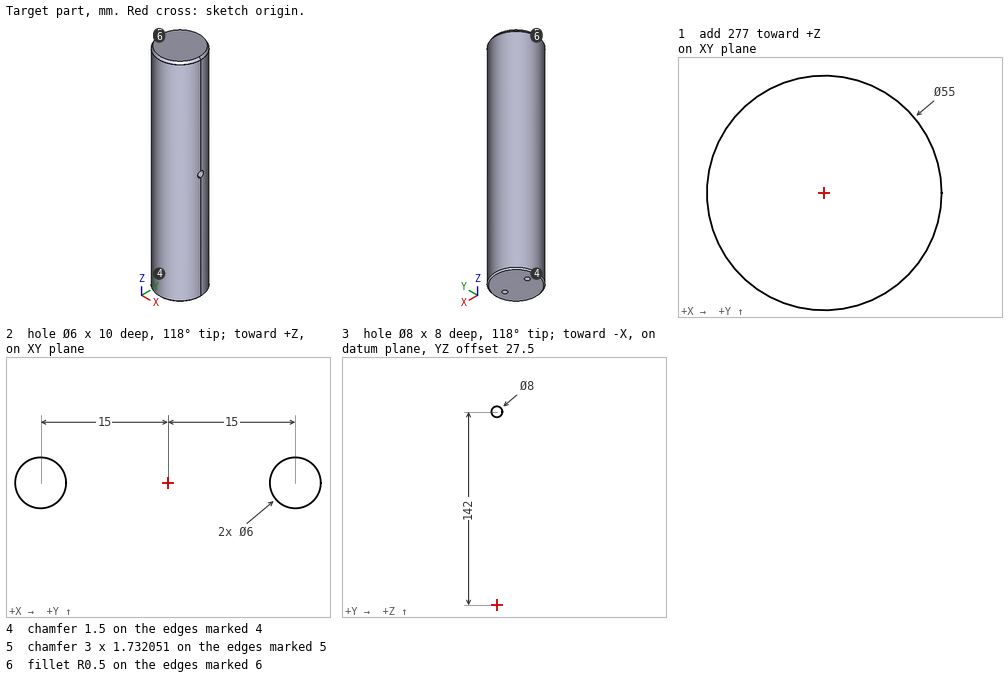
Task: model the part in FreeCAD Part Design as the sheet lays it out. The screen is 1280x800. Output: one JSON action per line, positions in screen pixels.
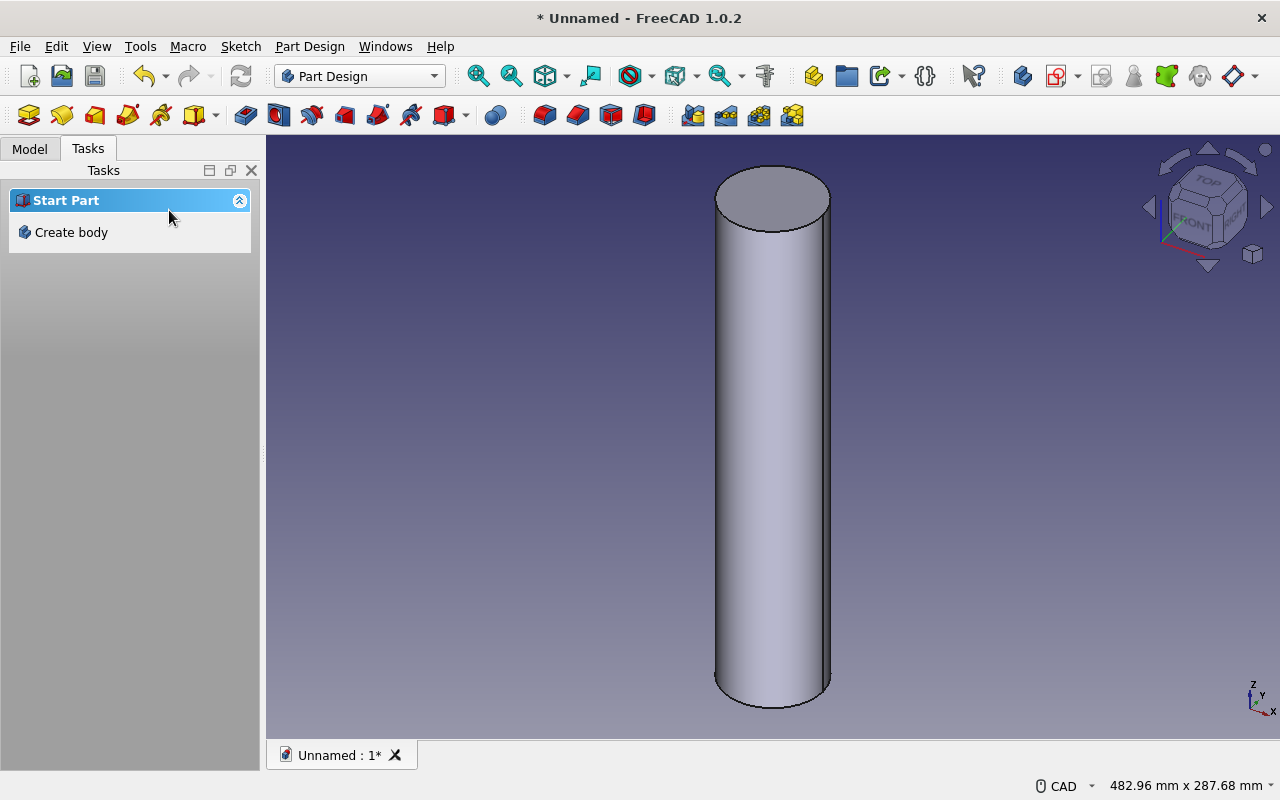
{"action": "left_click", "coordinate": [30, 148]}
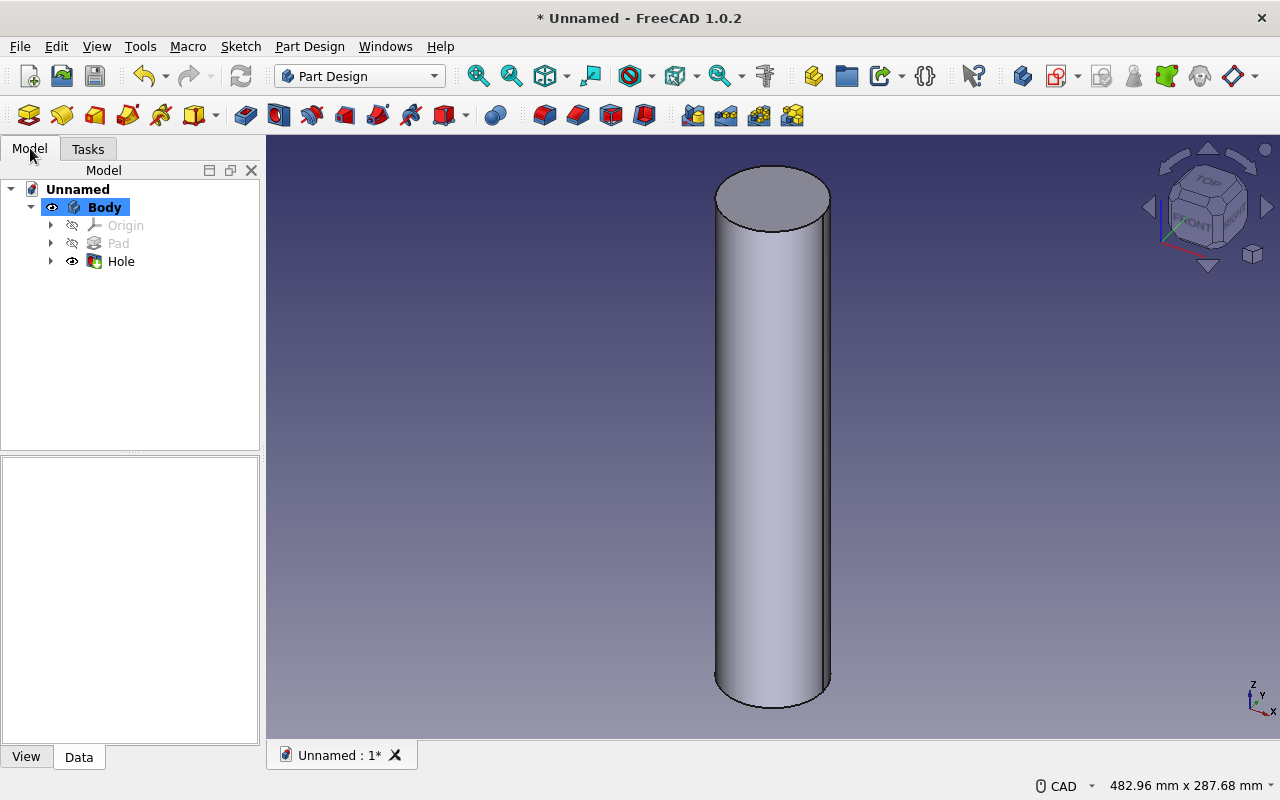
{"action": "left_click", "coordinate": [51, 225]}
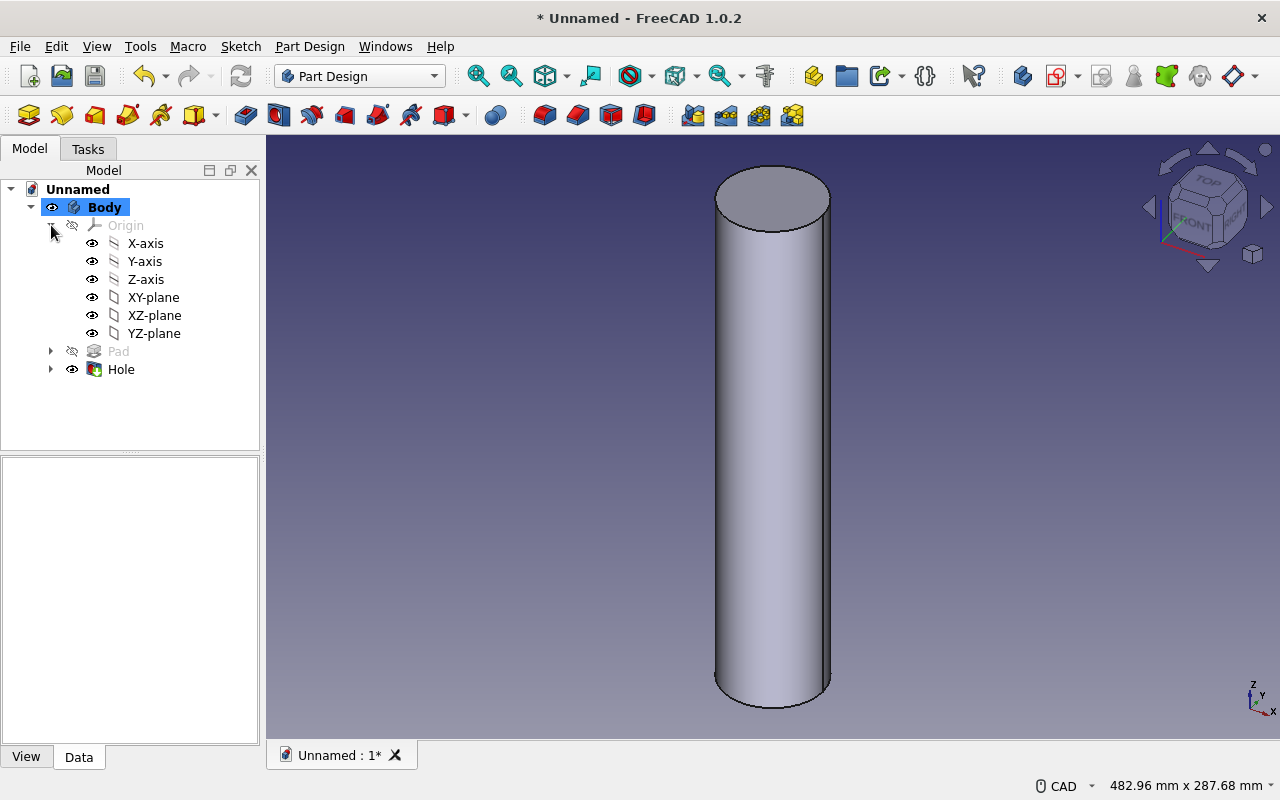
{"action": "left_click", "coordinate": [137, 333]}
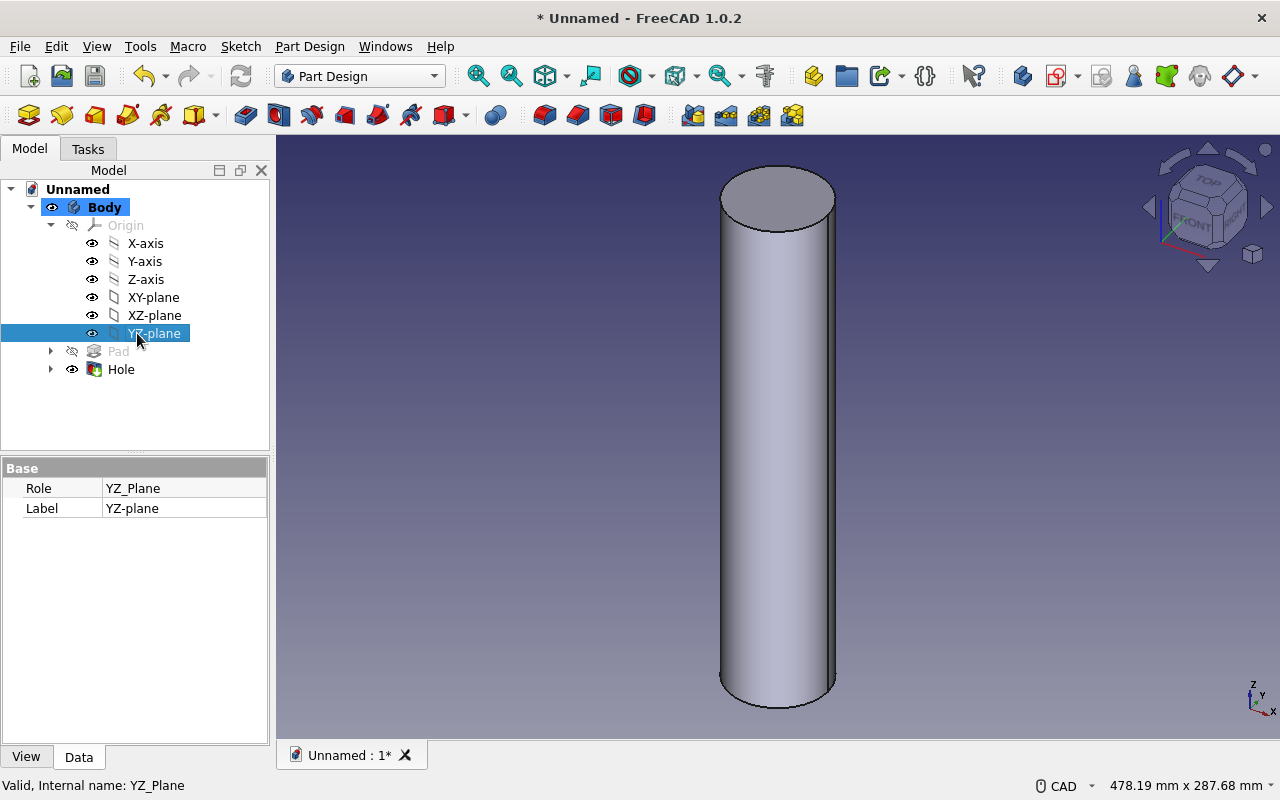
{"action": "left_click", "coordinate": [1232, 76]}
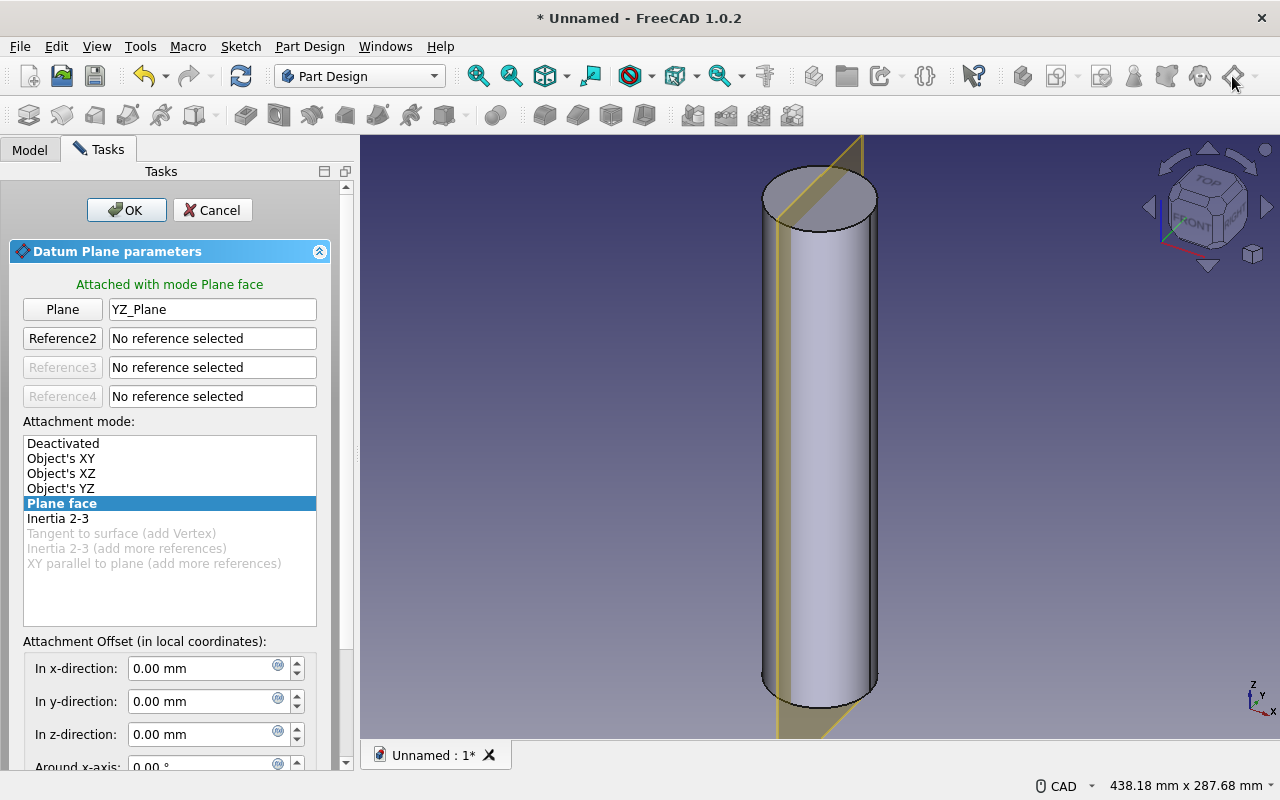
{"action": "triple_click", "coordinate": [210, 734]}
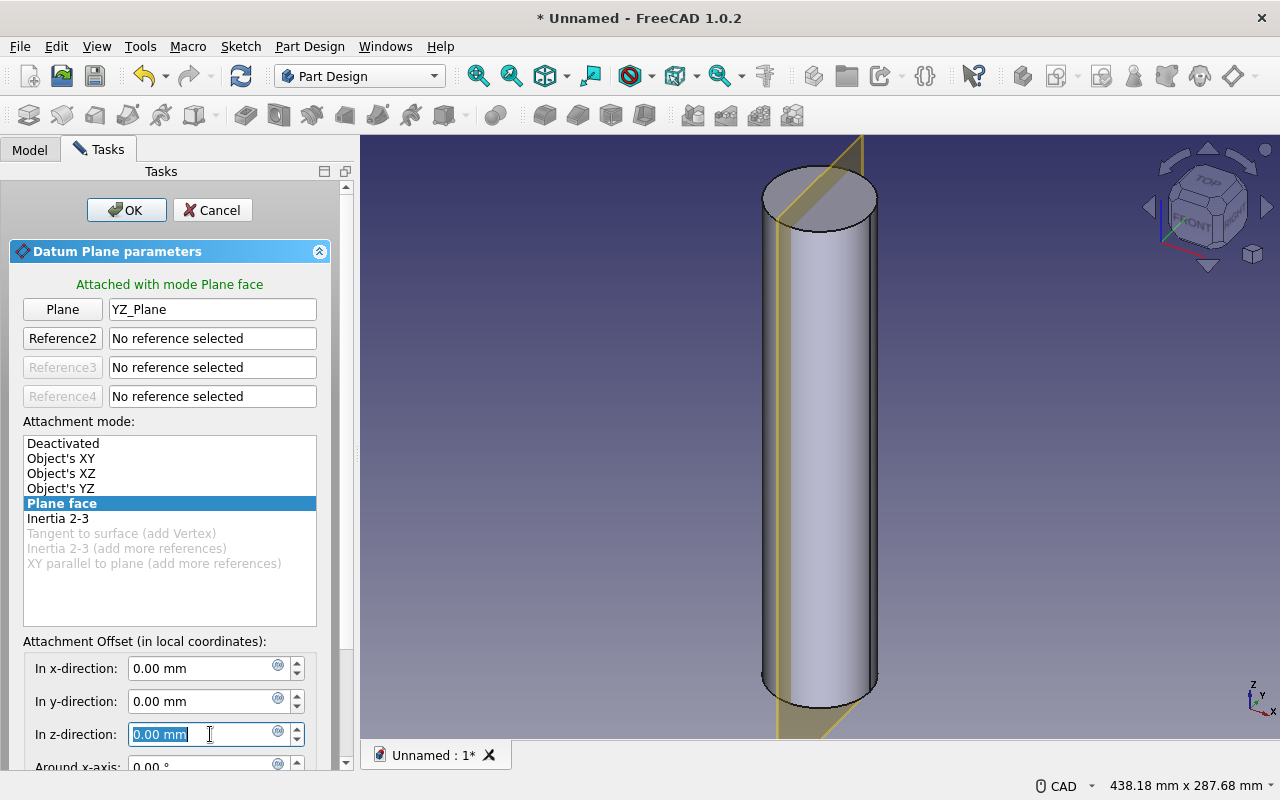
{"action": "type", "text": "27.5"}
{"action": "key", "text": "Tab"}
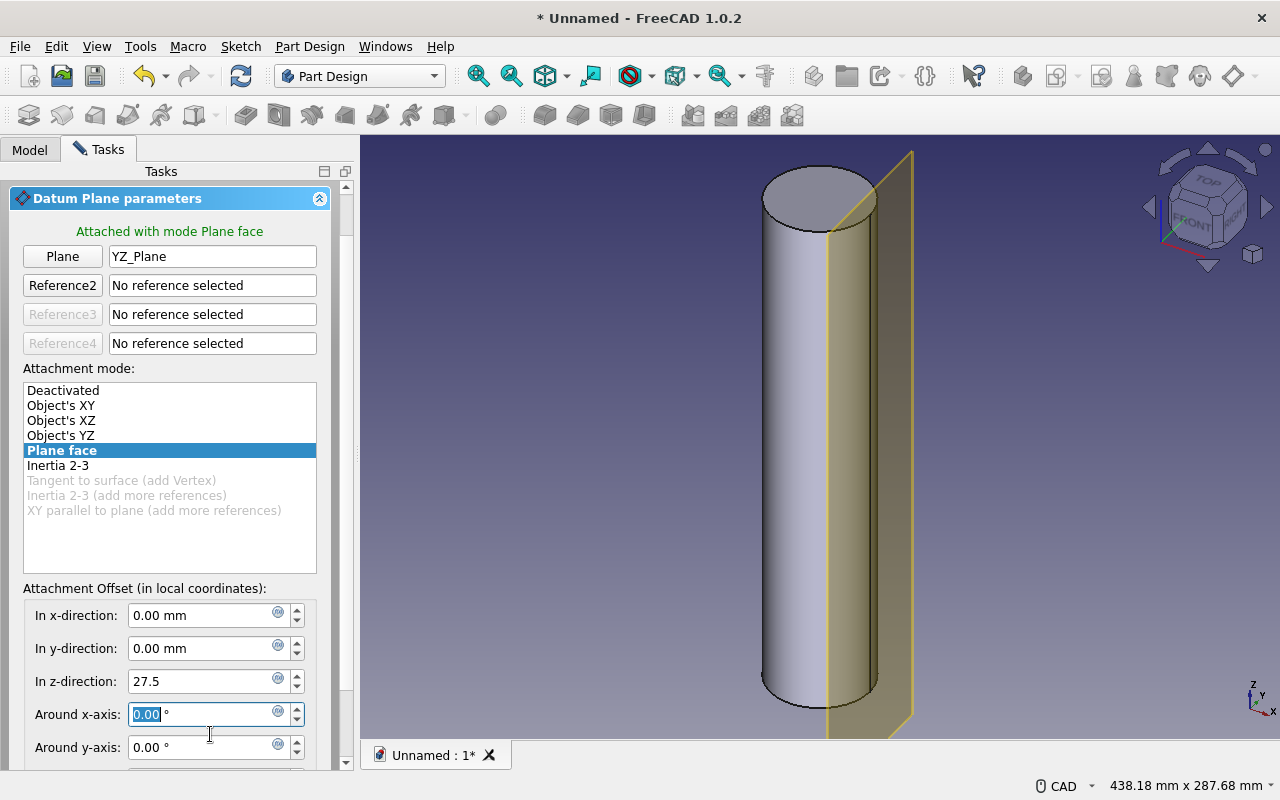
{"action": "scroll", "coordinate": [346, 476], "scroll_direction": "up", "scroll_amount": 2}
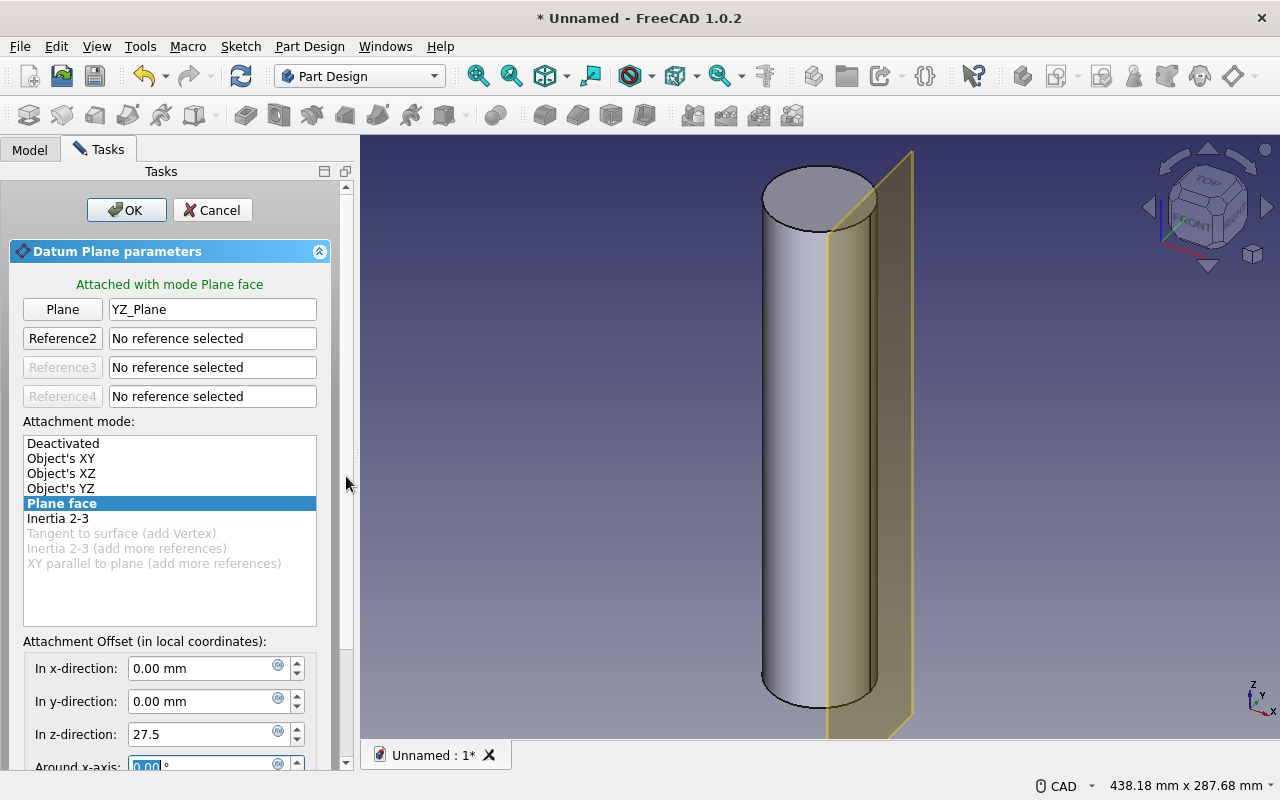
{"action": "left_click", "coordinate": [127, 210]}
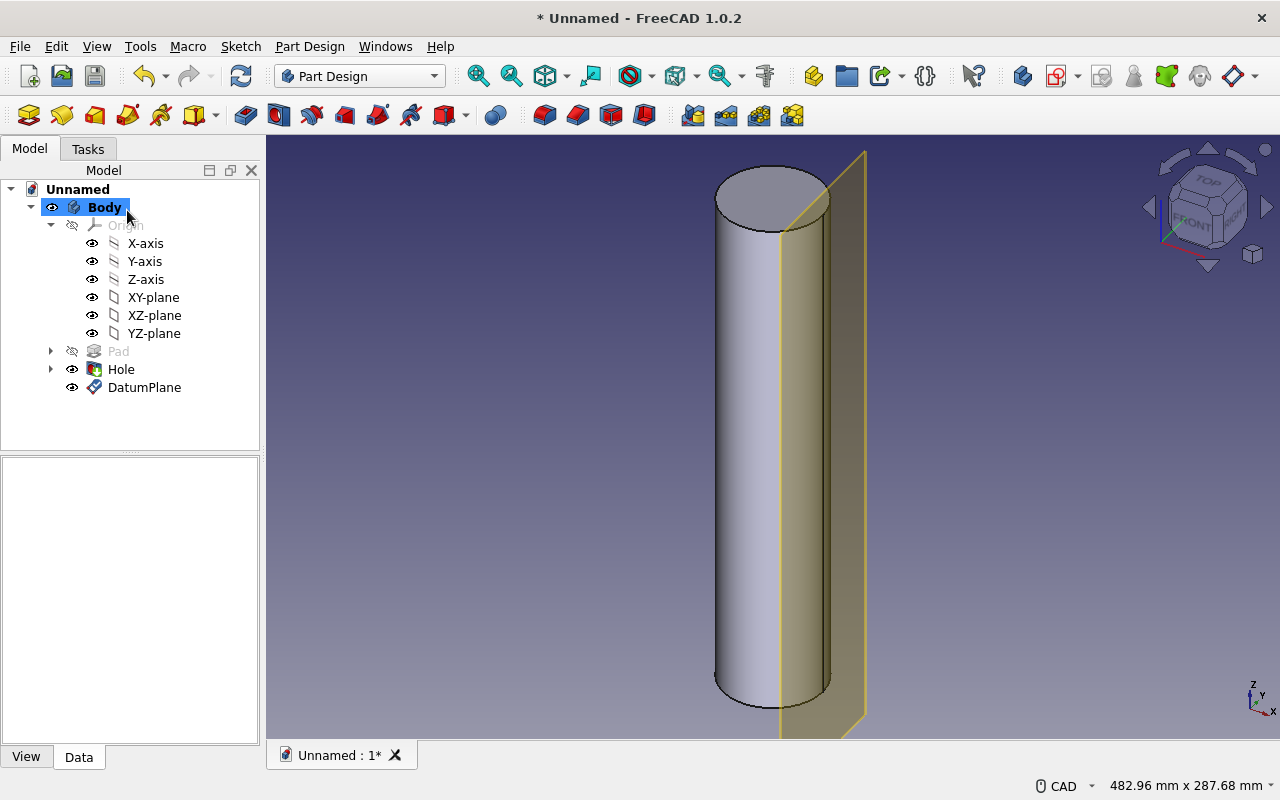
{"action": "left_click", "coordinate": [117, 387]}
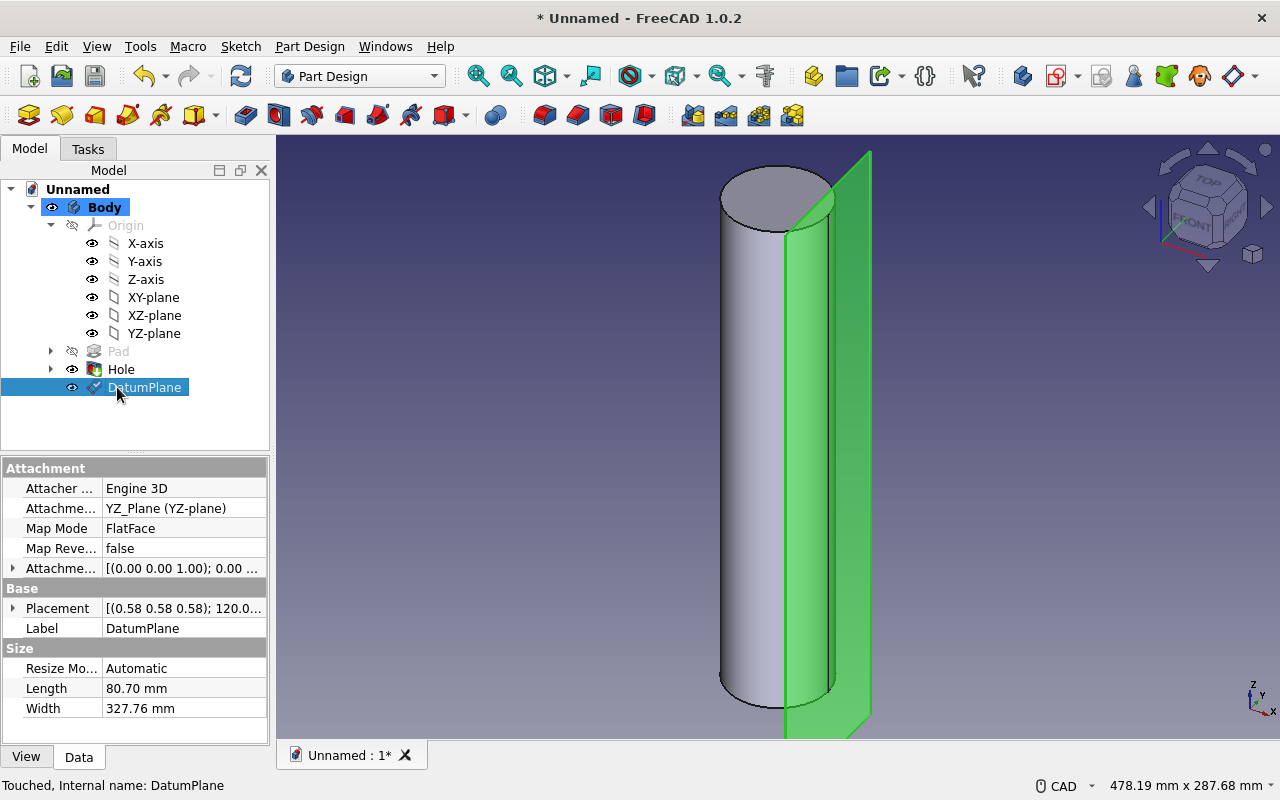
{"action": "left_click", "coordinate": [1056, 76]}